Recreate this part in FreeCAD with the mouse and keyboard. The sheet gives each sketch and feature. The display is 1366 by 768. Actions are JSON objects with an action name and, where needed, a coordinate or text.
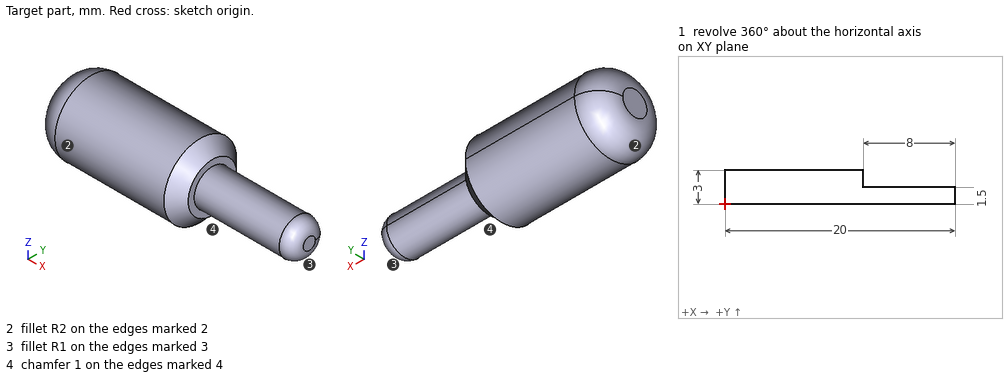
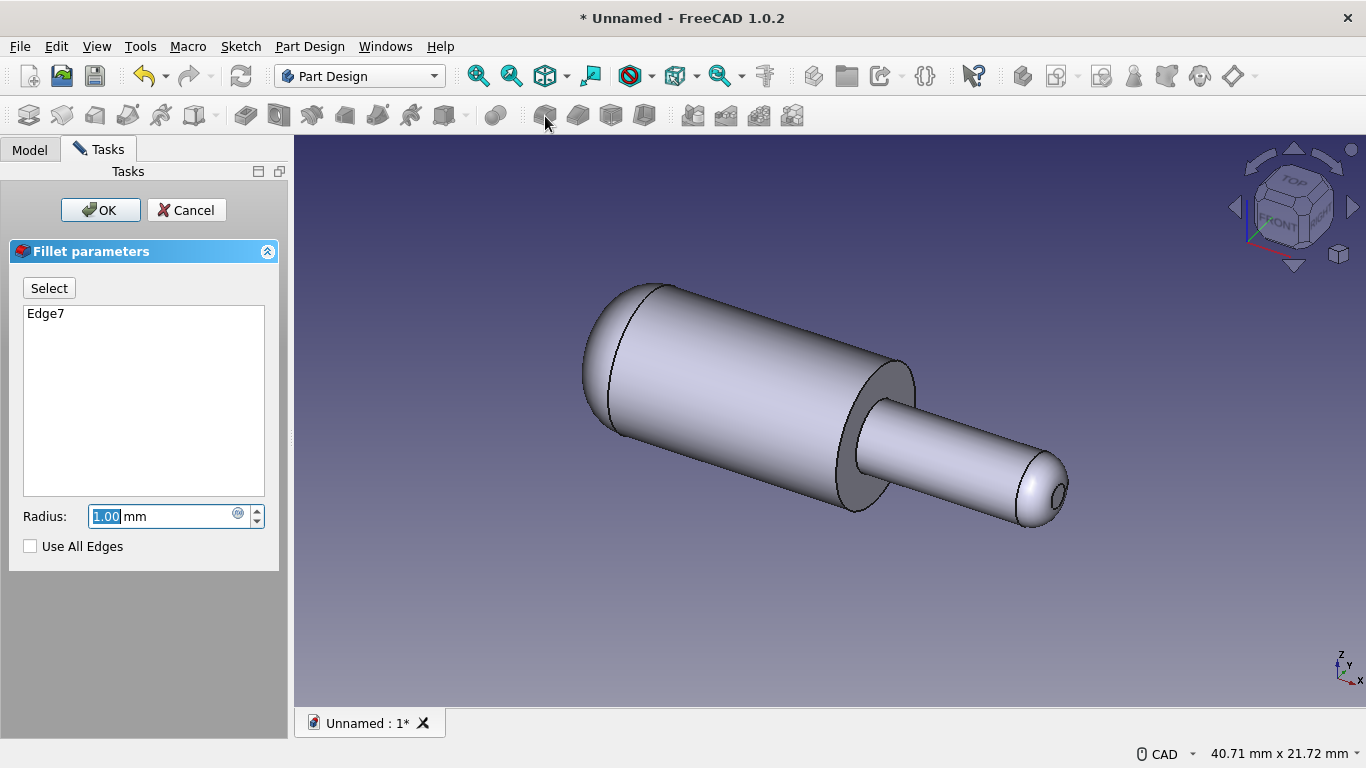
{"action": "type", "text": "1"}
{"action": "key", "text": "Tab"}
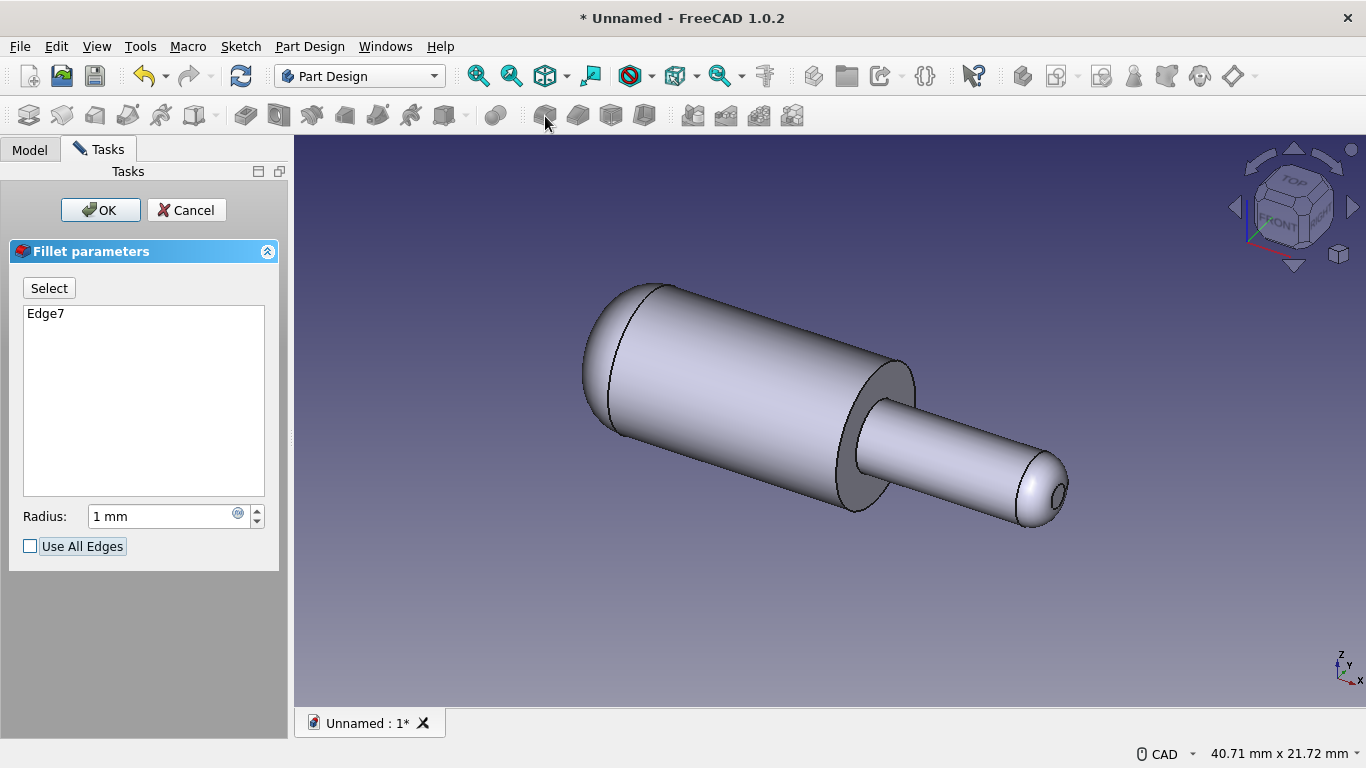
{"action": "left_click", "coordinate": [101, 210]}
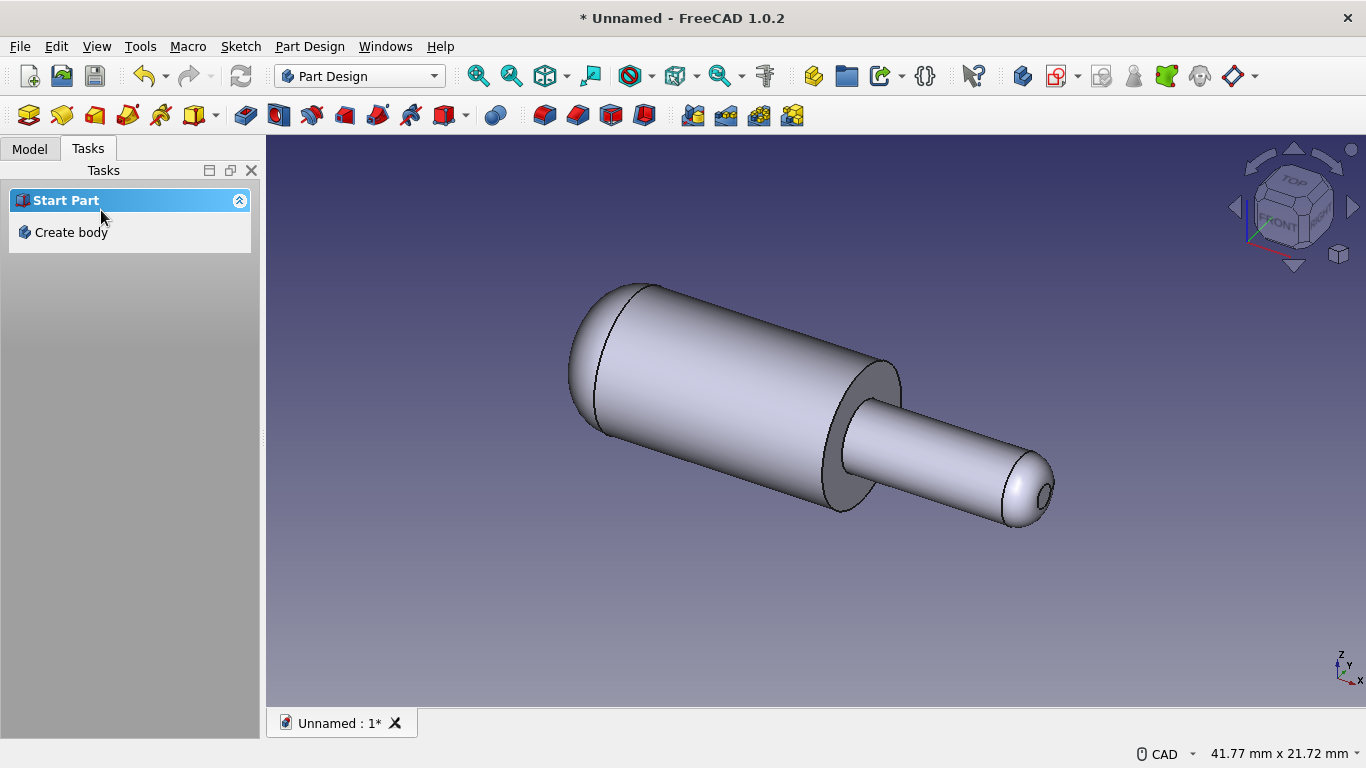
{"action": "left_click", "coordinate": [822, 474]}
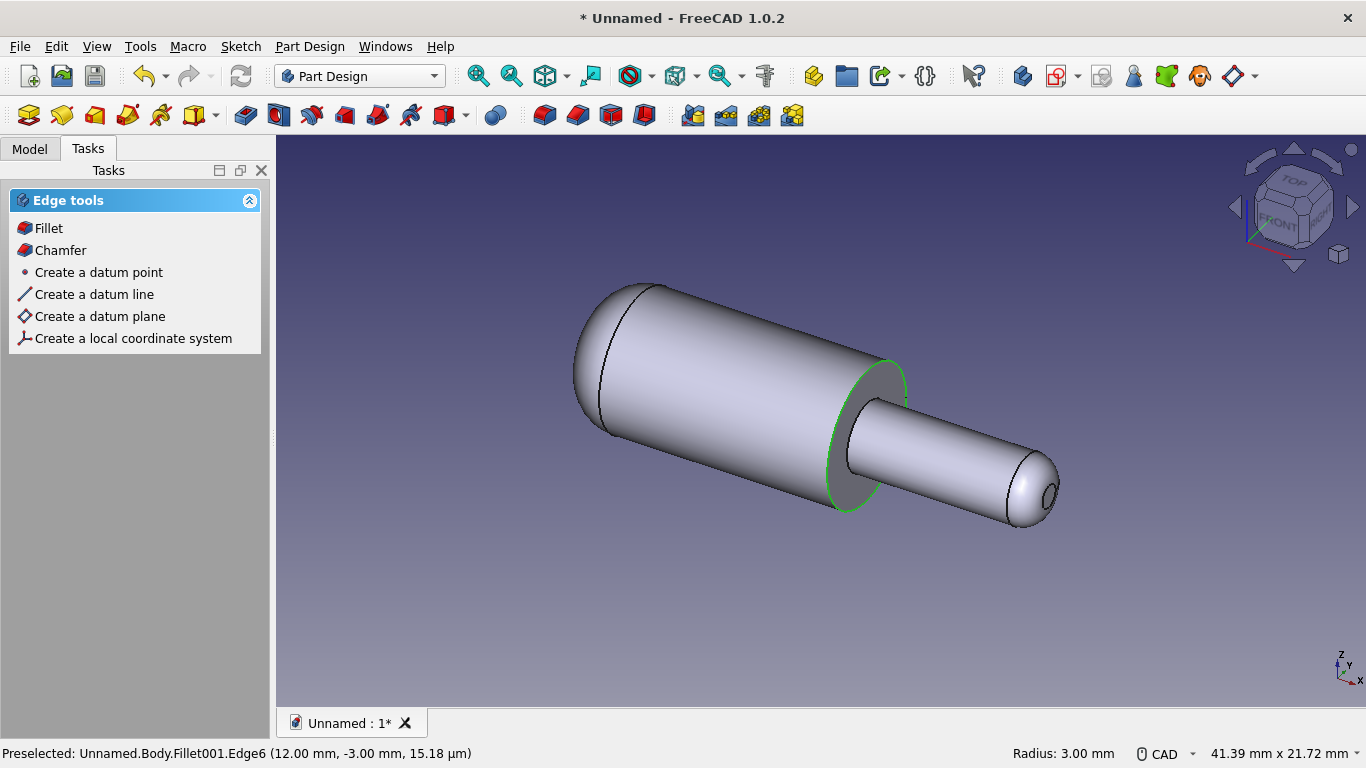
{"action": "left_click", "coordinate": [578, 116]}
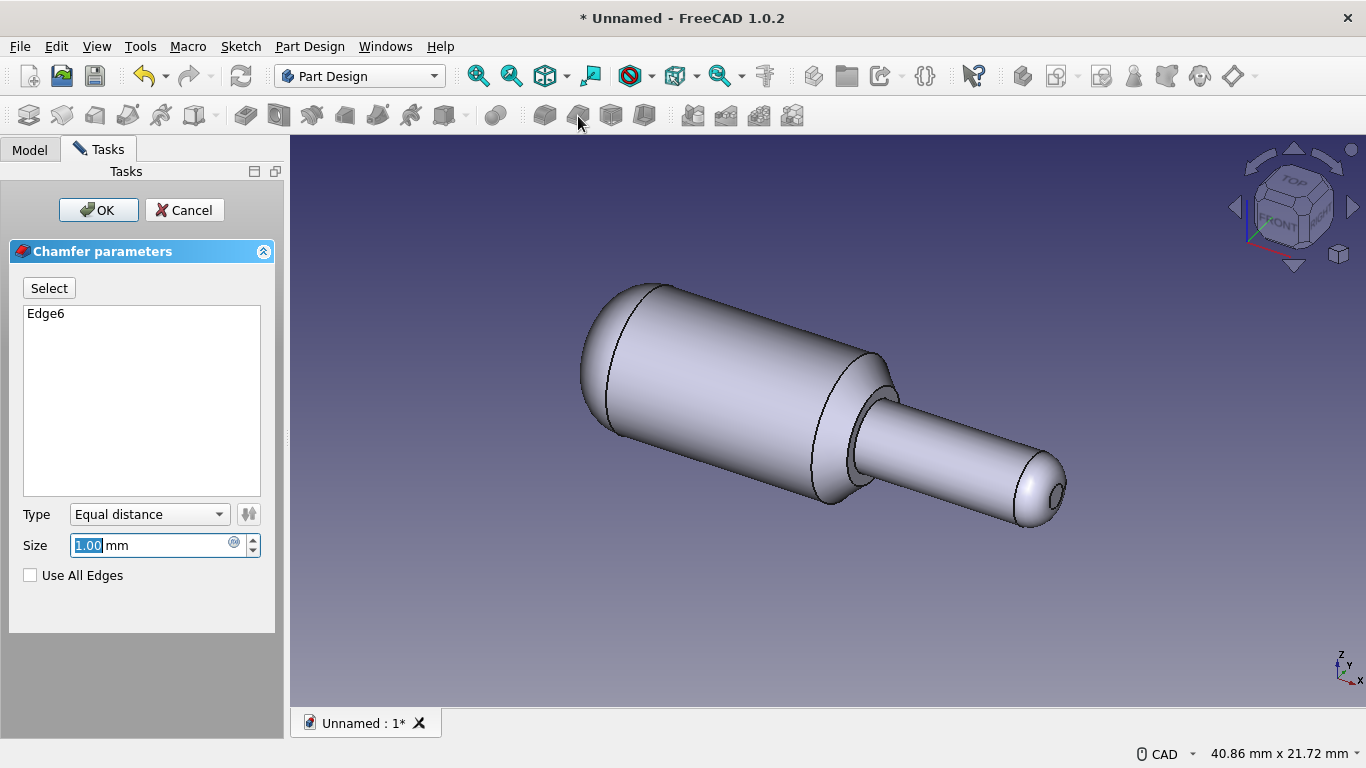
{"action": "type", "text": "1"}
{"action": "key", "text": "Tab"}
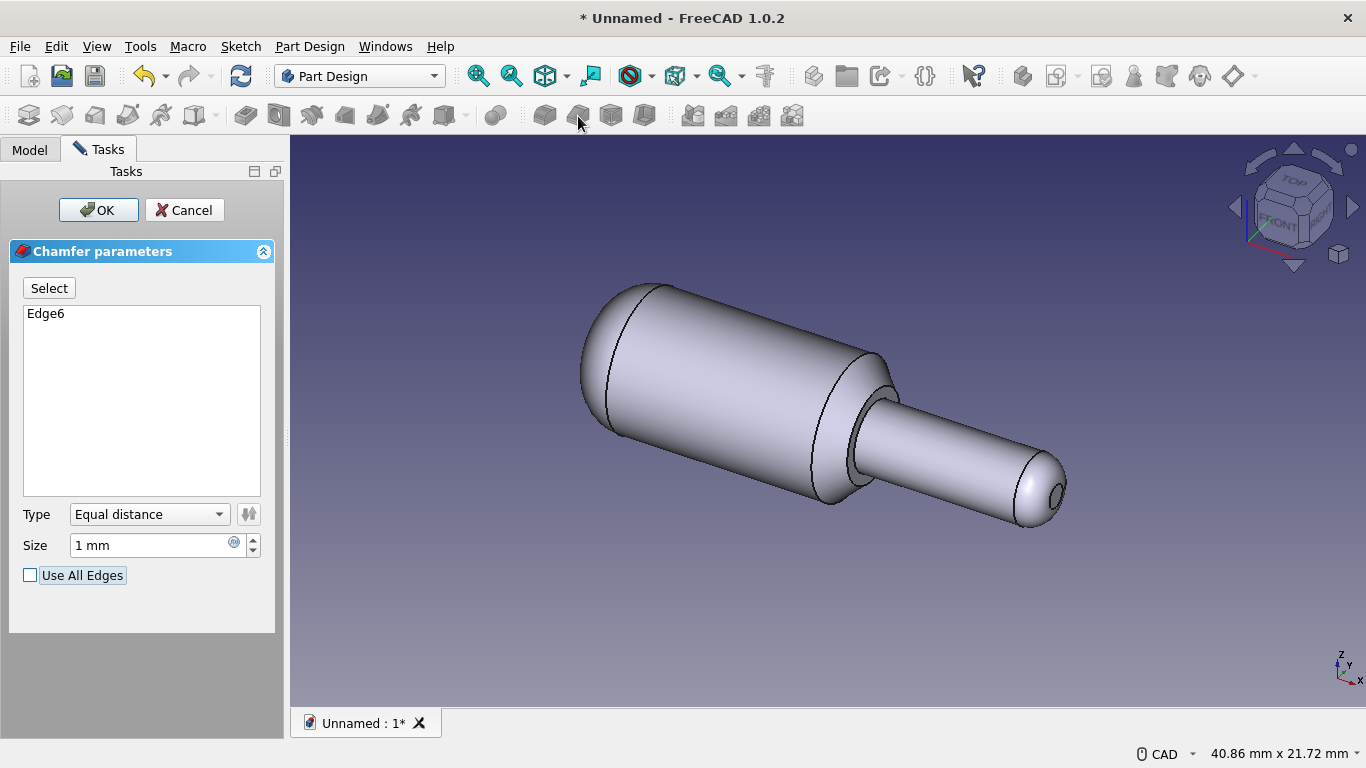
{"action": "left_click", "coordinate": [99, 210]}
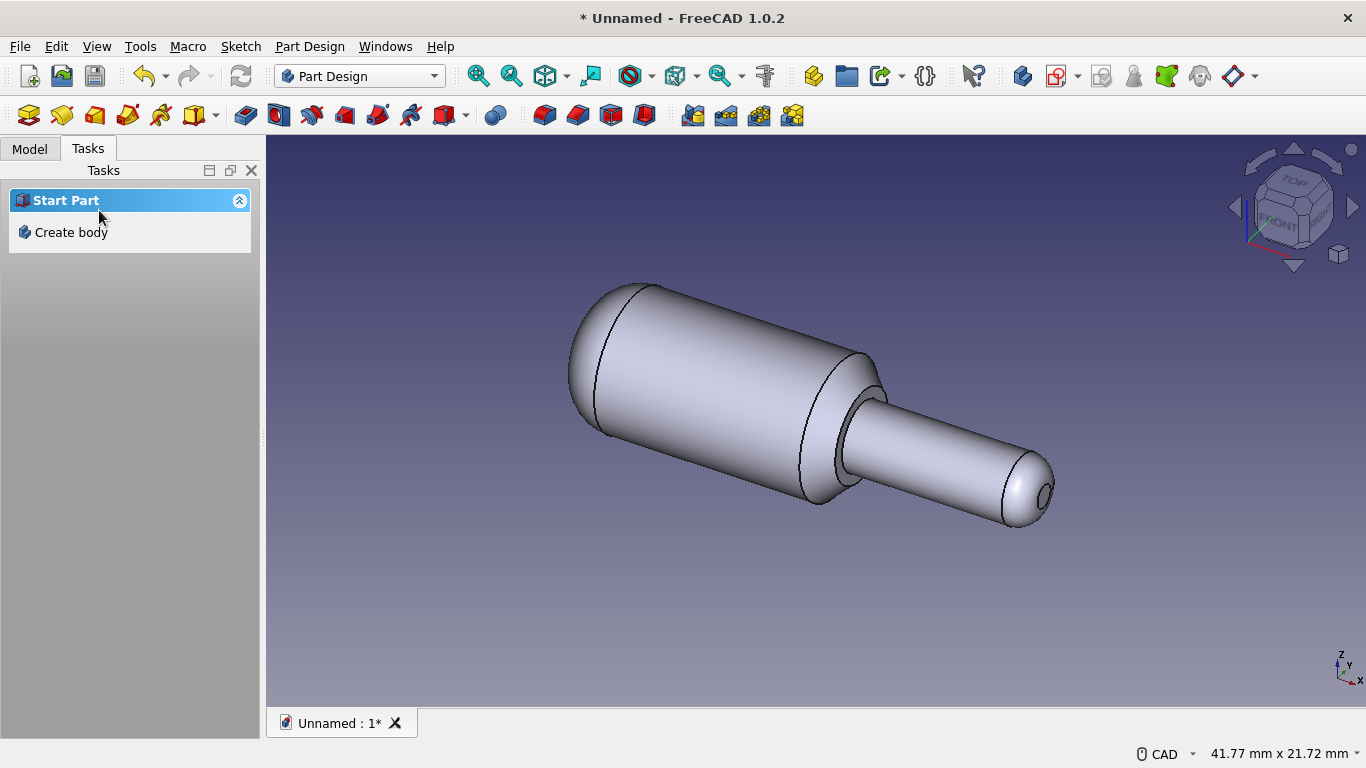
{"action": "key", "text": "0"}